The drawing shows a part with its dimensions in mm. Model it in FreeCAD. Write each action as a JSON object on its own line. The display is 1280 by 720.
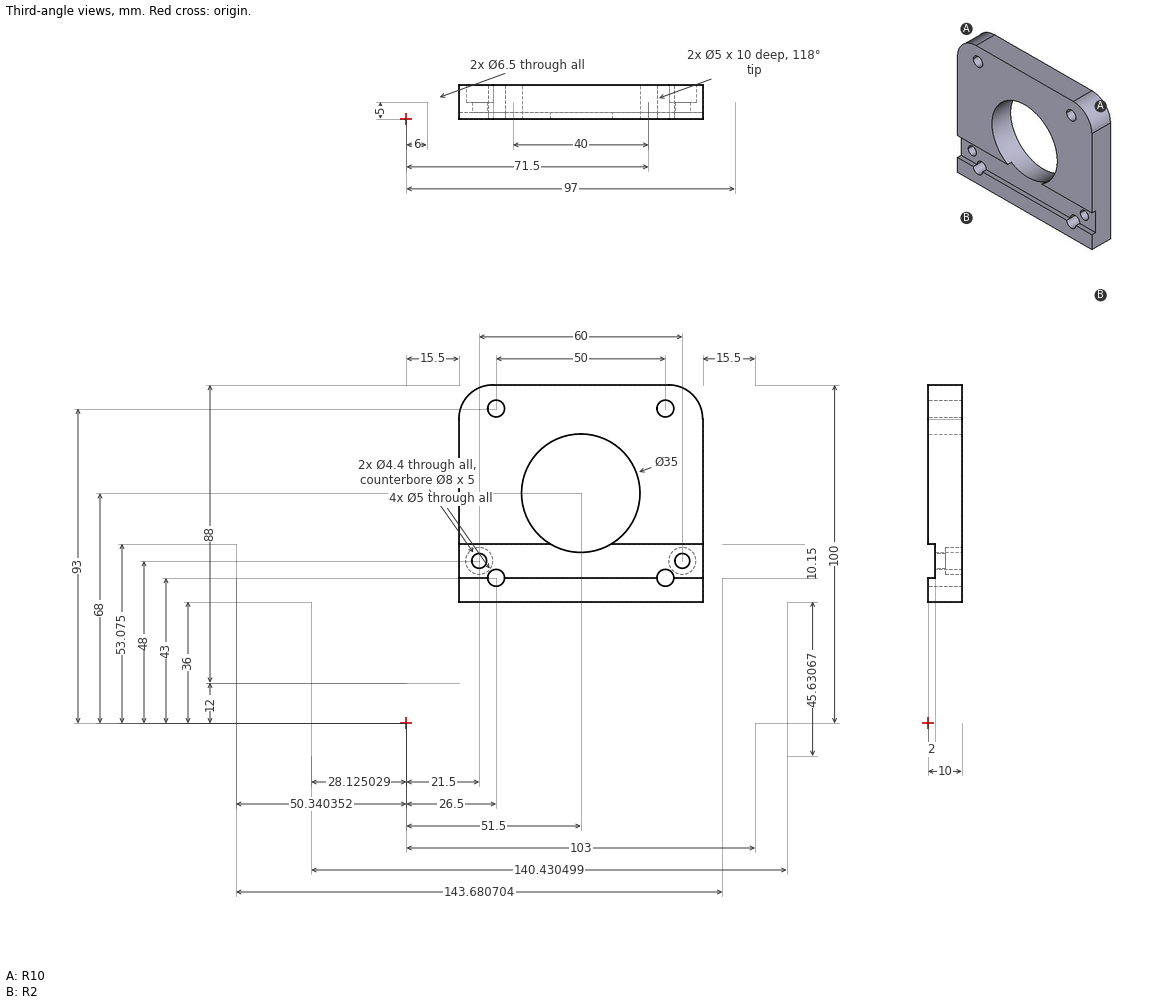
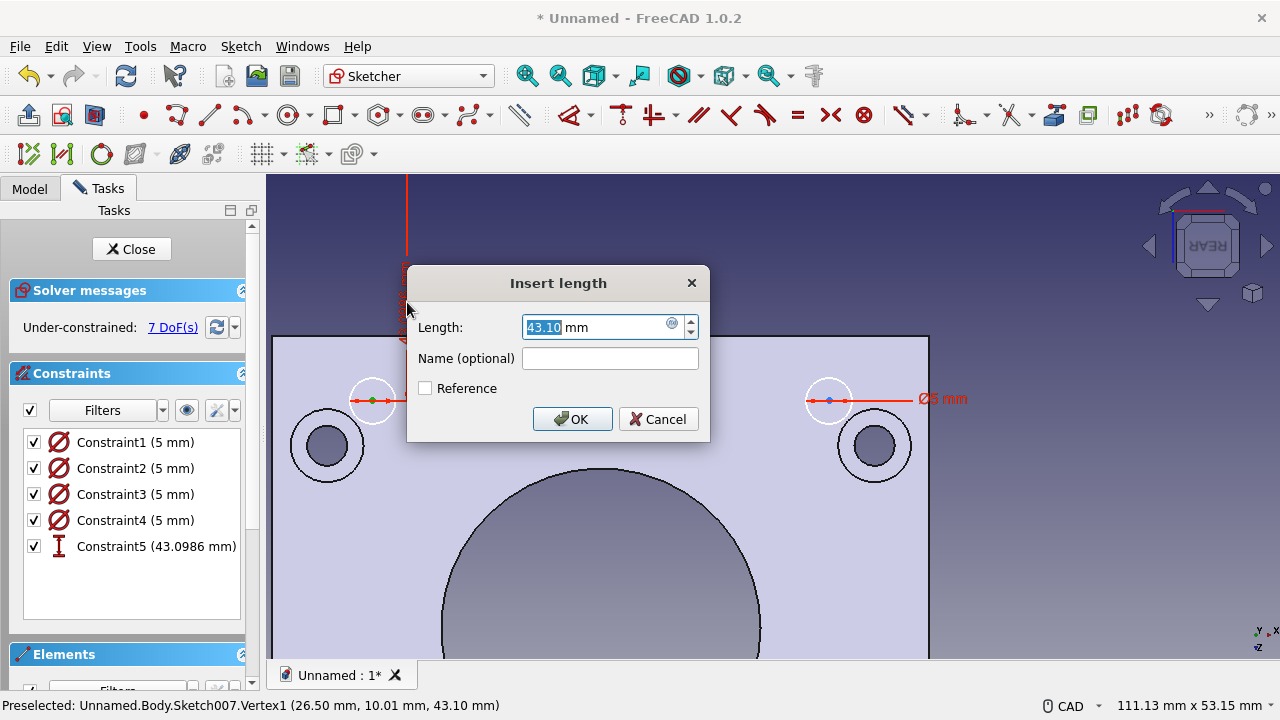
{"action": "type", "text": "43"}
{"action": "key", "text": "Return"}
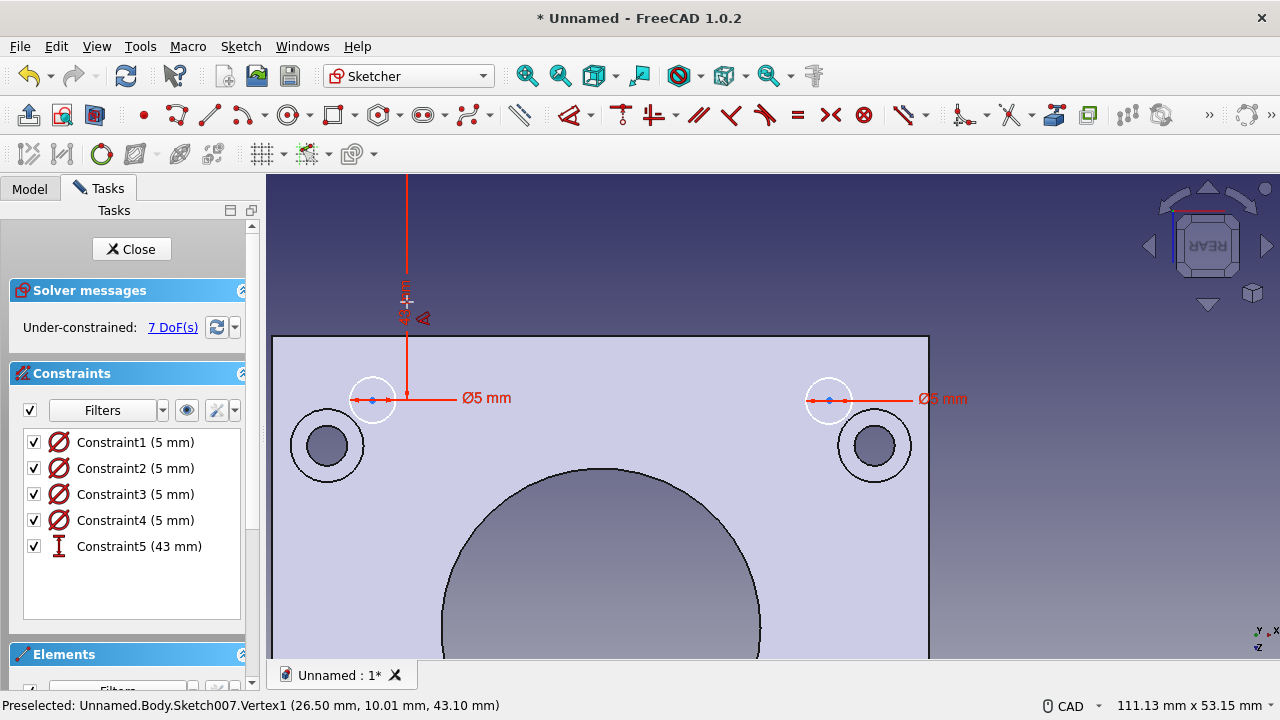
{"action": "scroll", "coordinate": [829, 401], "scroll_direction": "down", "scroll_amount": 5}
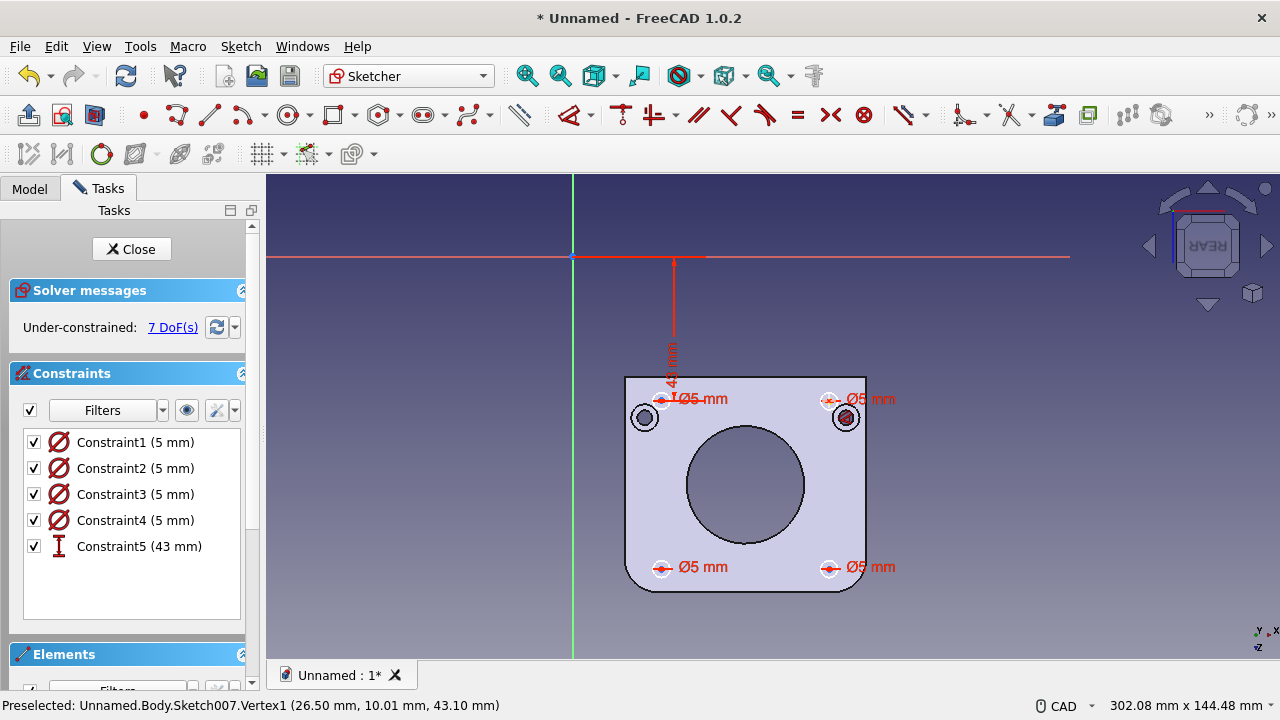
{"action": "left_click", "coordinate": [662, 569]}
{"action": "left_click", "coordinate": [539, 413]}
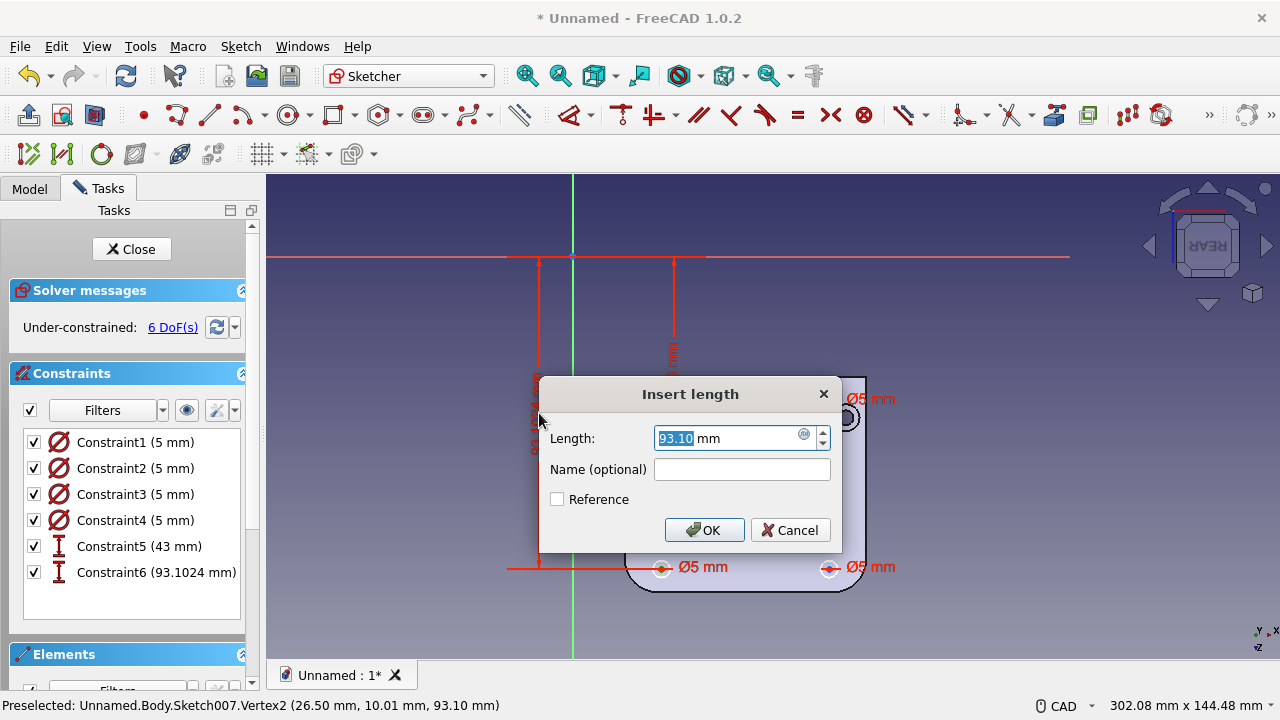
{"action": "type", "text": "93"}
{"action": "key", "text": "Return"}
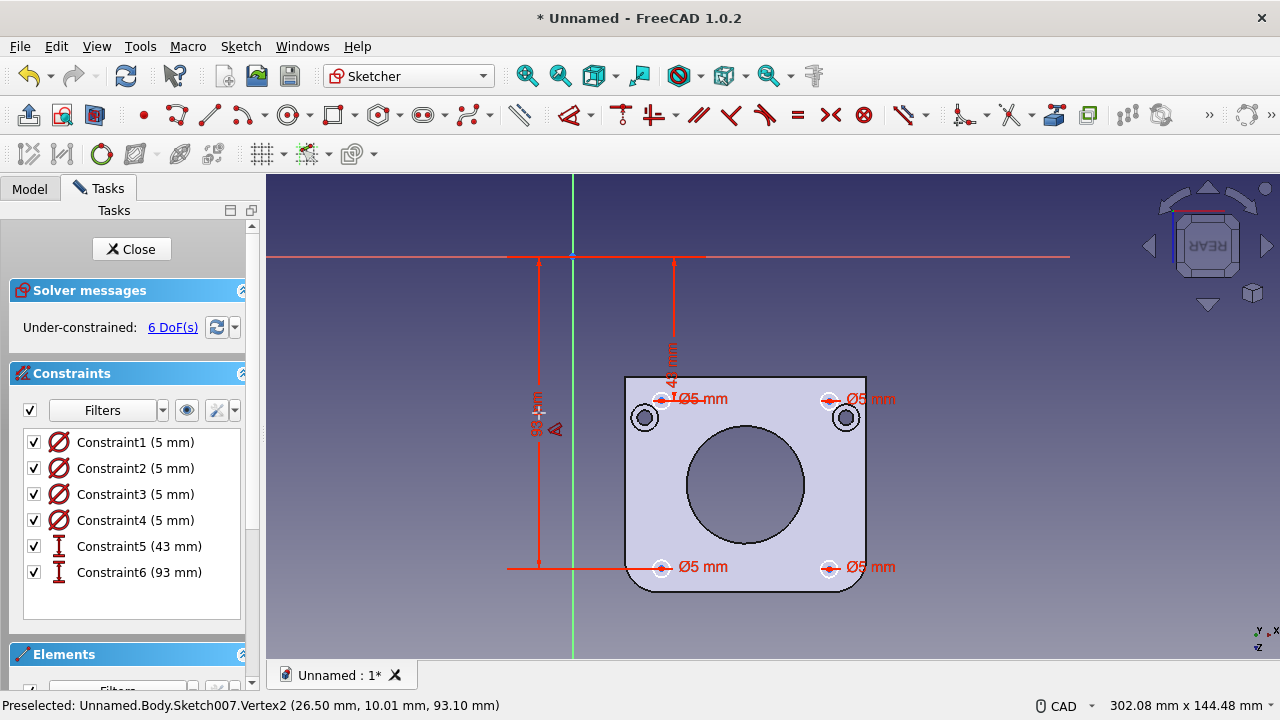
{"action": "left_click", "coordinate": [829, 569]}
{"action": "left_click", "coordinate": [539, 341]}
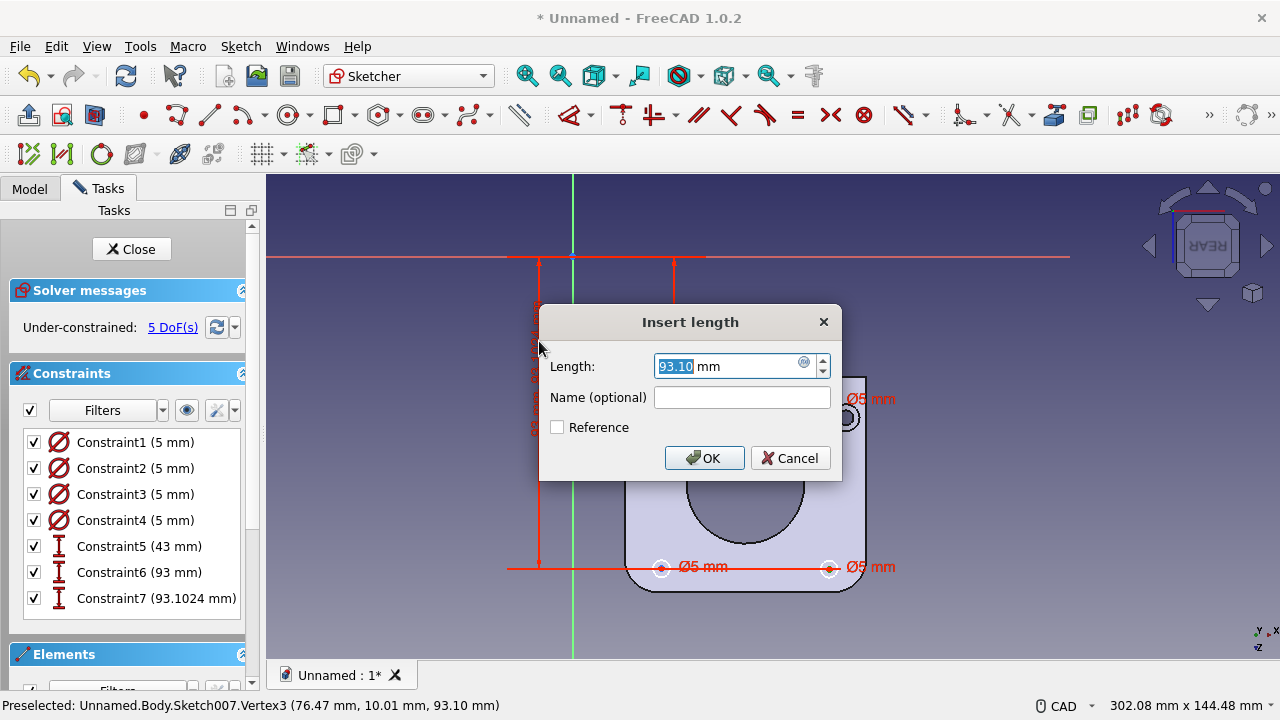
{"action": "type", "text": "93"}
{"action": "key", "text": "Return"}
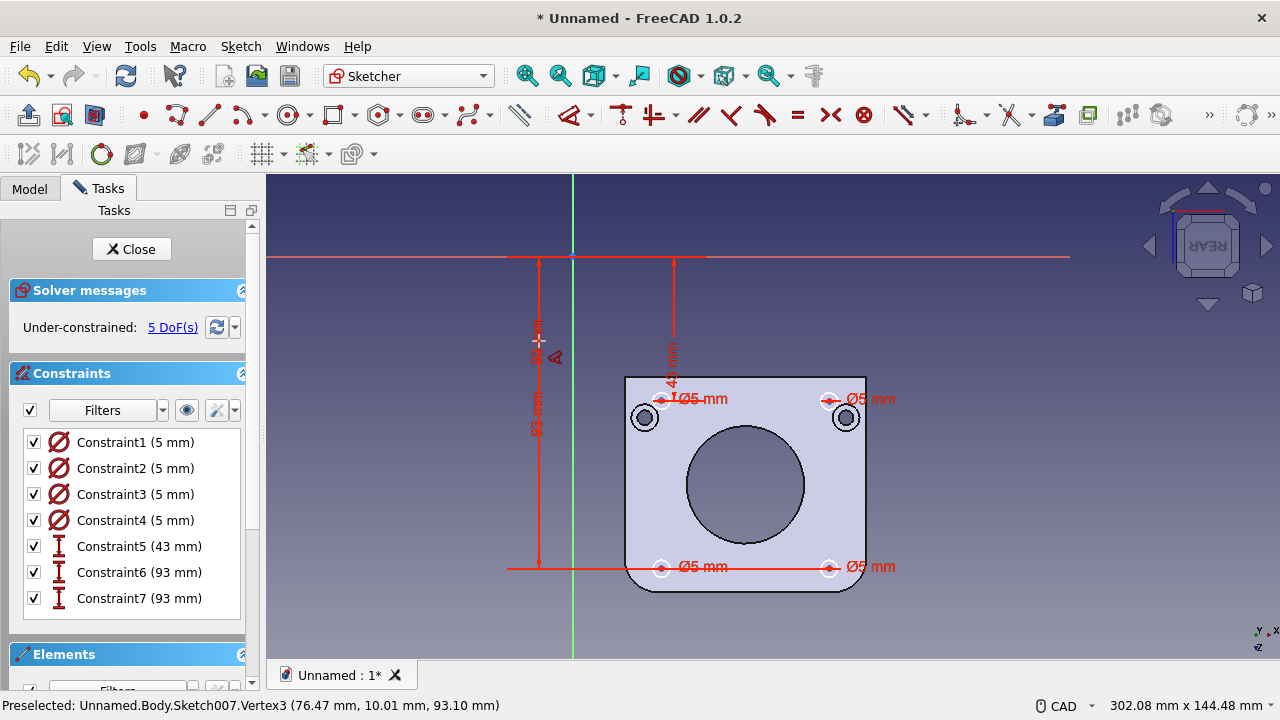
{"action": "left_click", "coordinate": [829, 401]}
{"action": "left_click", "coordinate": [539, 296]}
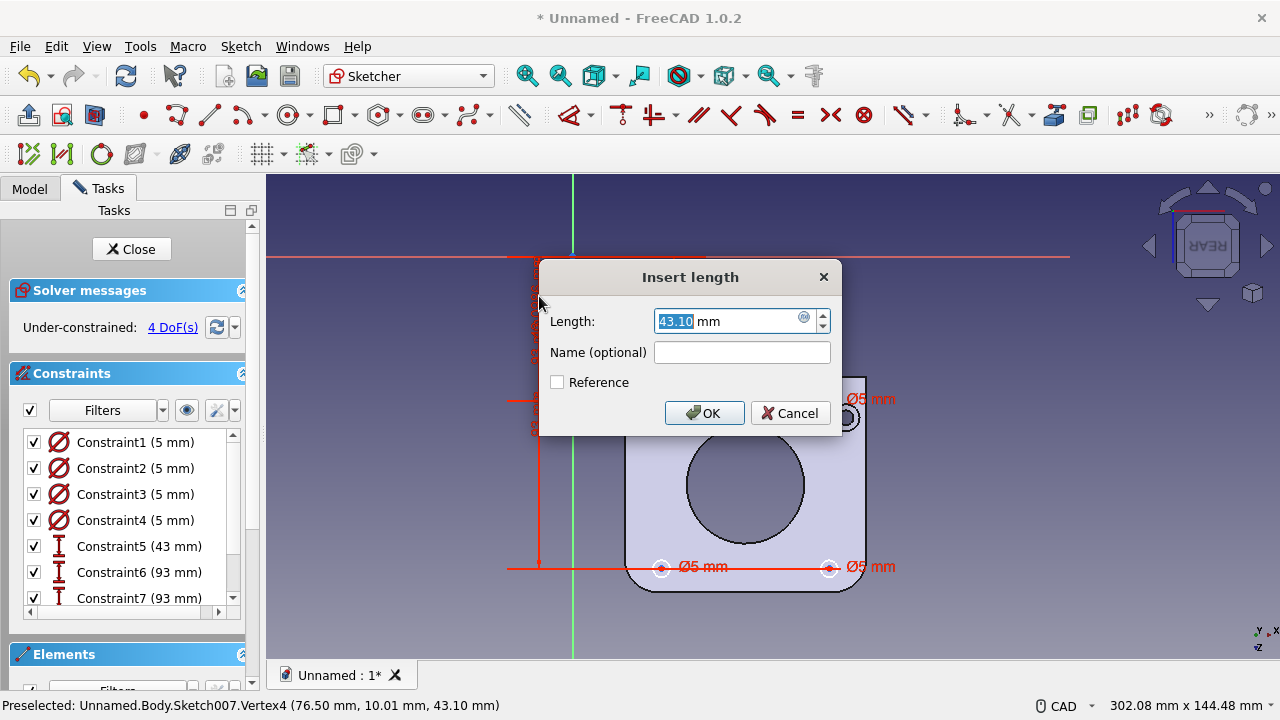
{"action": "type", "text": "43"}
{"action": "key", "text": "Return"}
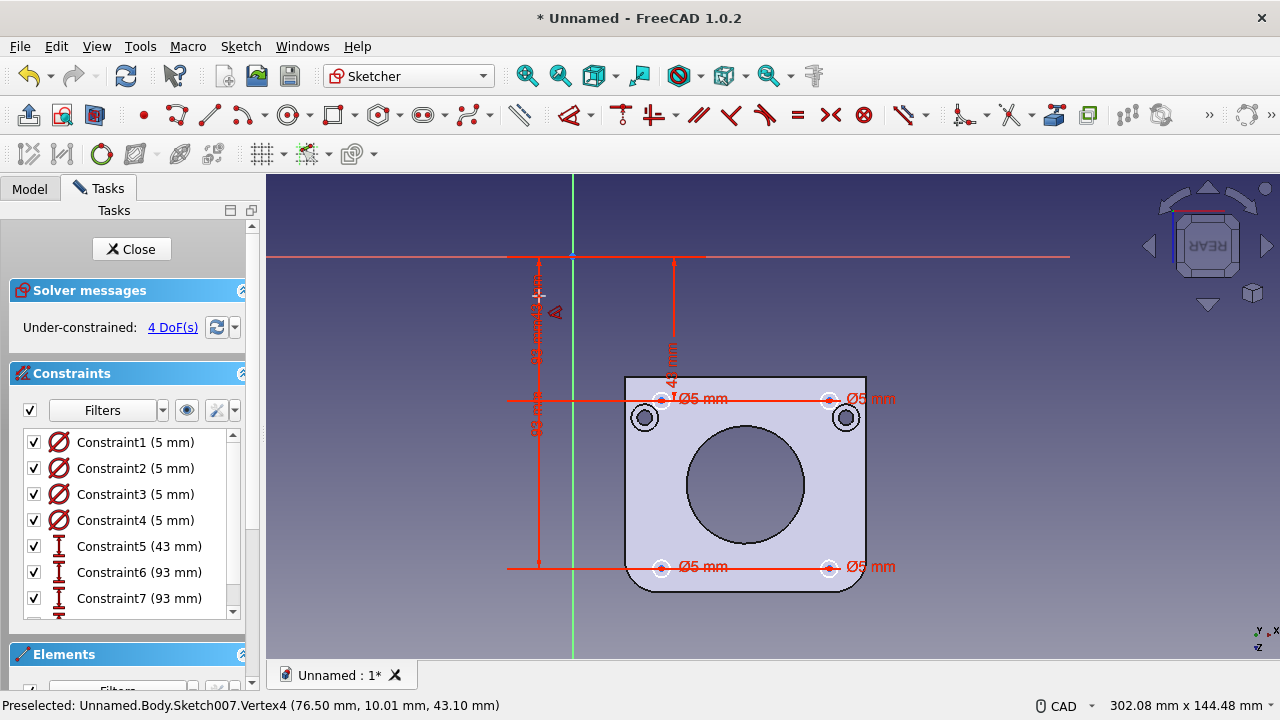
{"action": "left_click", "coordinate": [662, 569]}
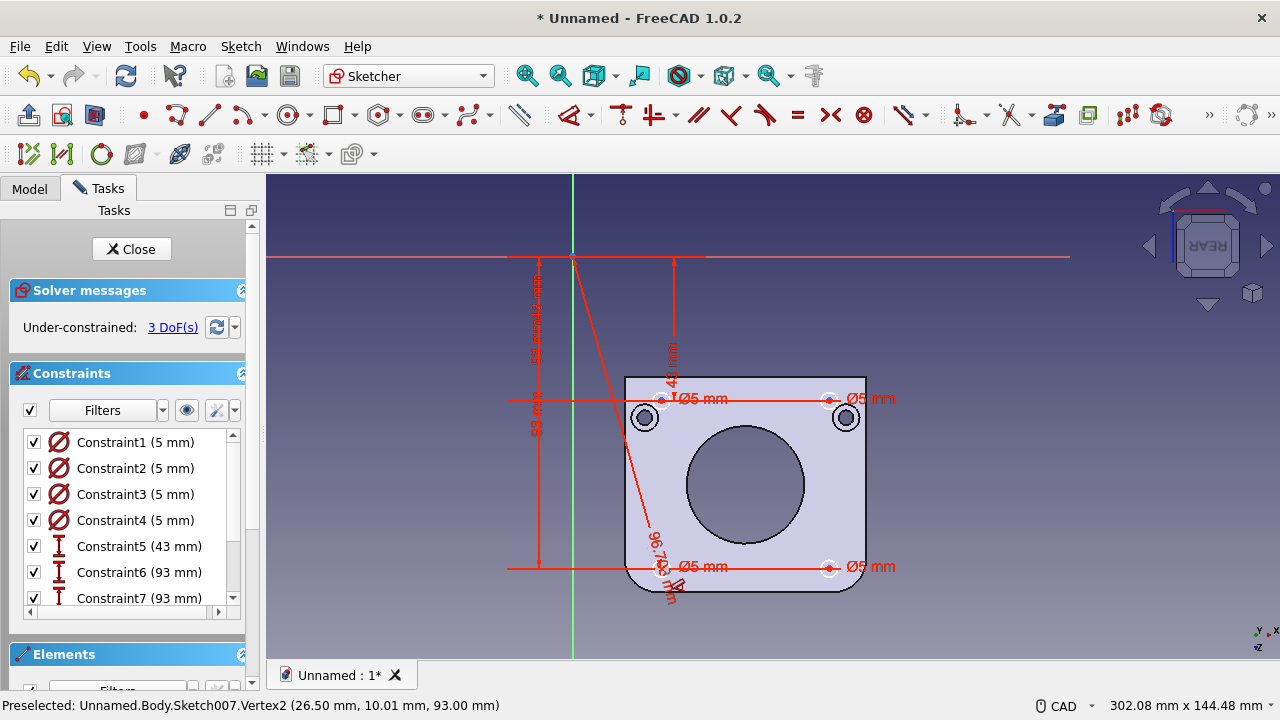
{"action": "left_click", "coordinate": [829, 569]}
{"action": "left_click", "coordinate": [745, 603]}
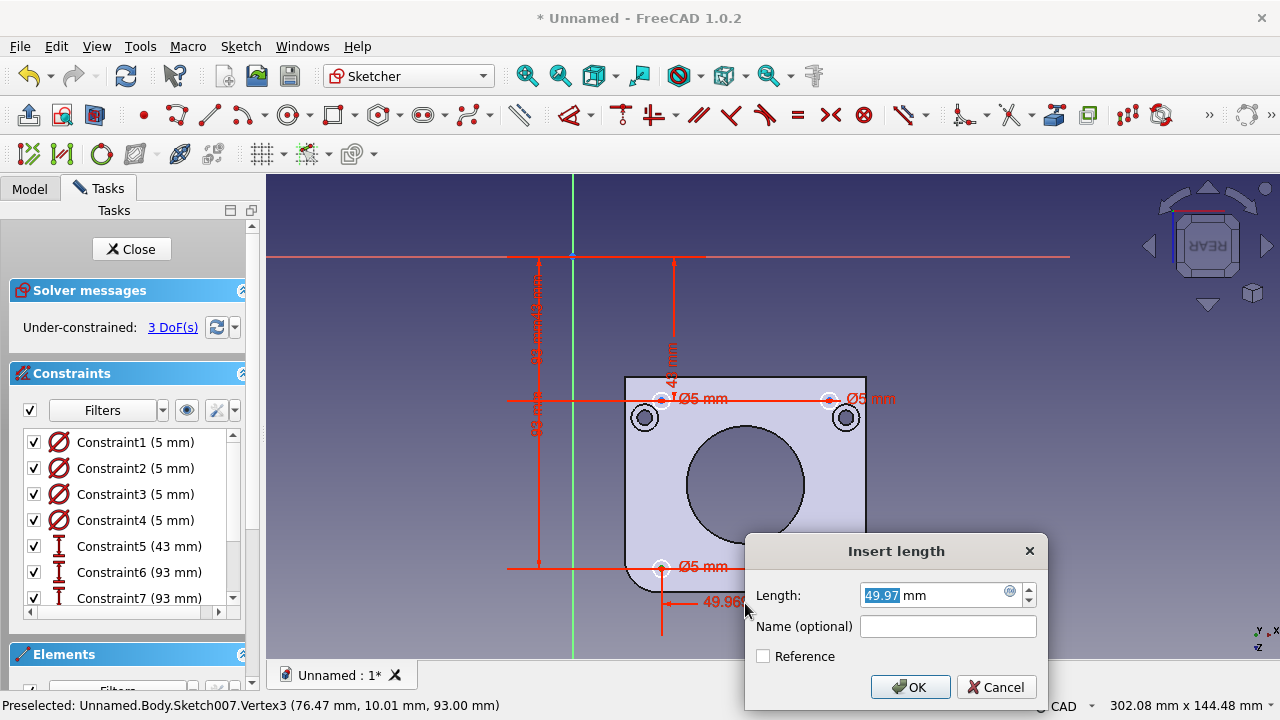
{"action": "type", "text": "50"}
{"action": "key", "text": "Return"}